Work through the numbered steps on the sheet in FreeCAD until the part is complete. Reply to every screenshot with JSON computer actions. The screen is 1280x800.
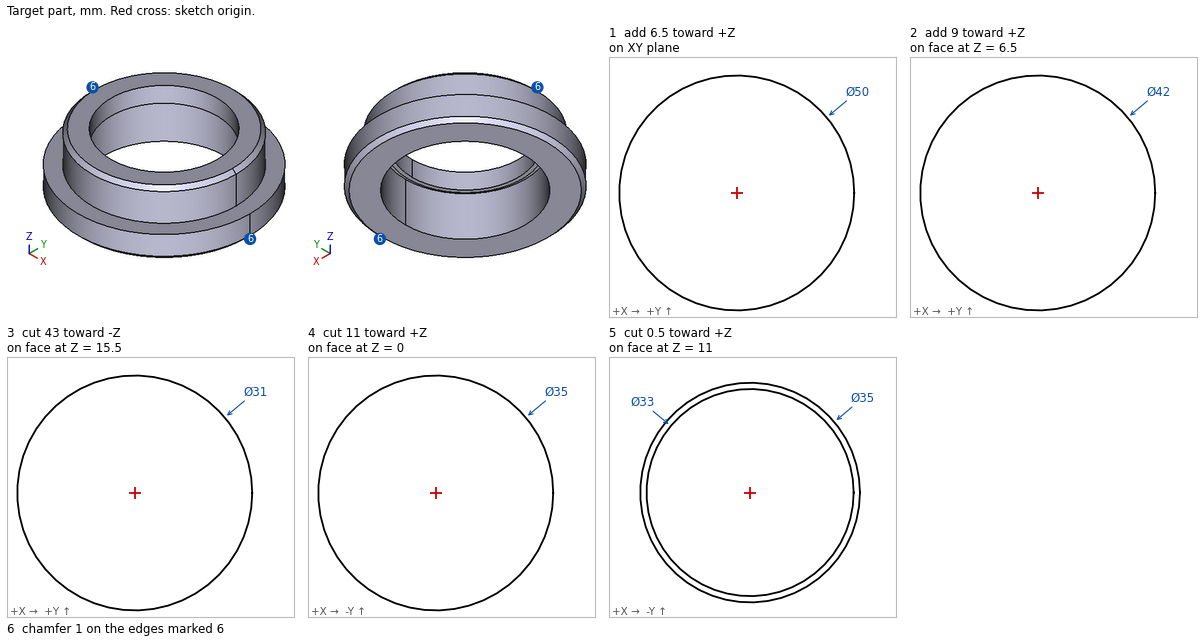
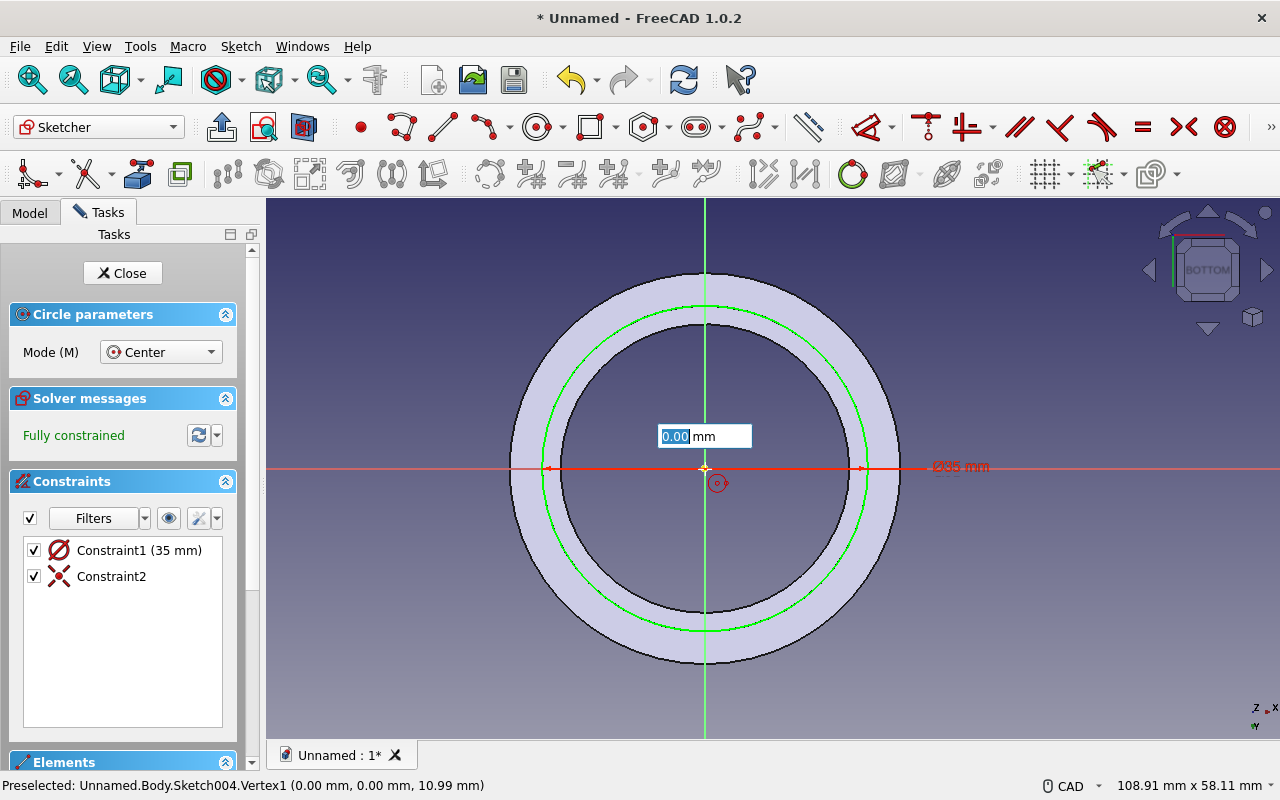
{"action": "scroll", "coordinate": [814, 360], "scroll_direction": "up", "scroll_amount": 3}
{"action": "mouse_move", "coordinate": [813, 360]}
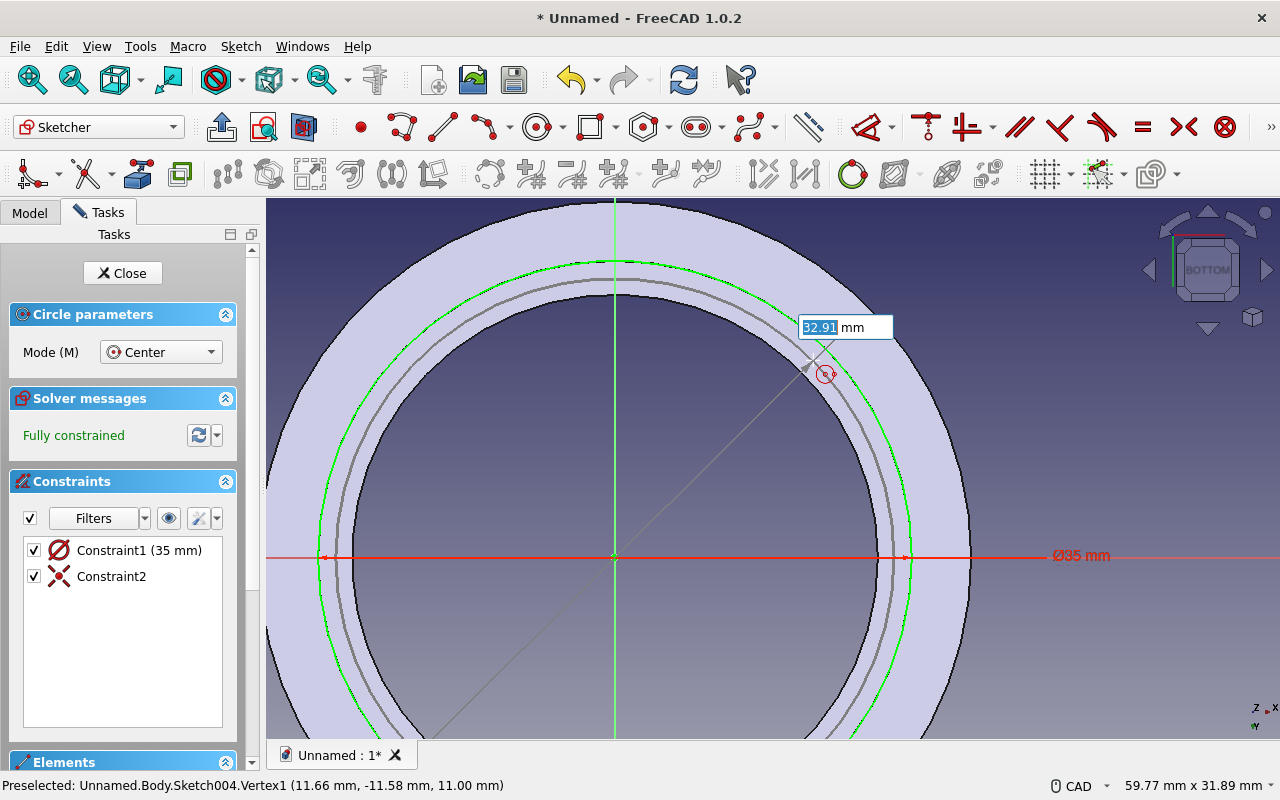
{"action": "type", "text": "33"}
{"action": "key", "text": "Return"}
{"action": "key", "text": "Escape"}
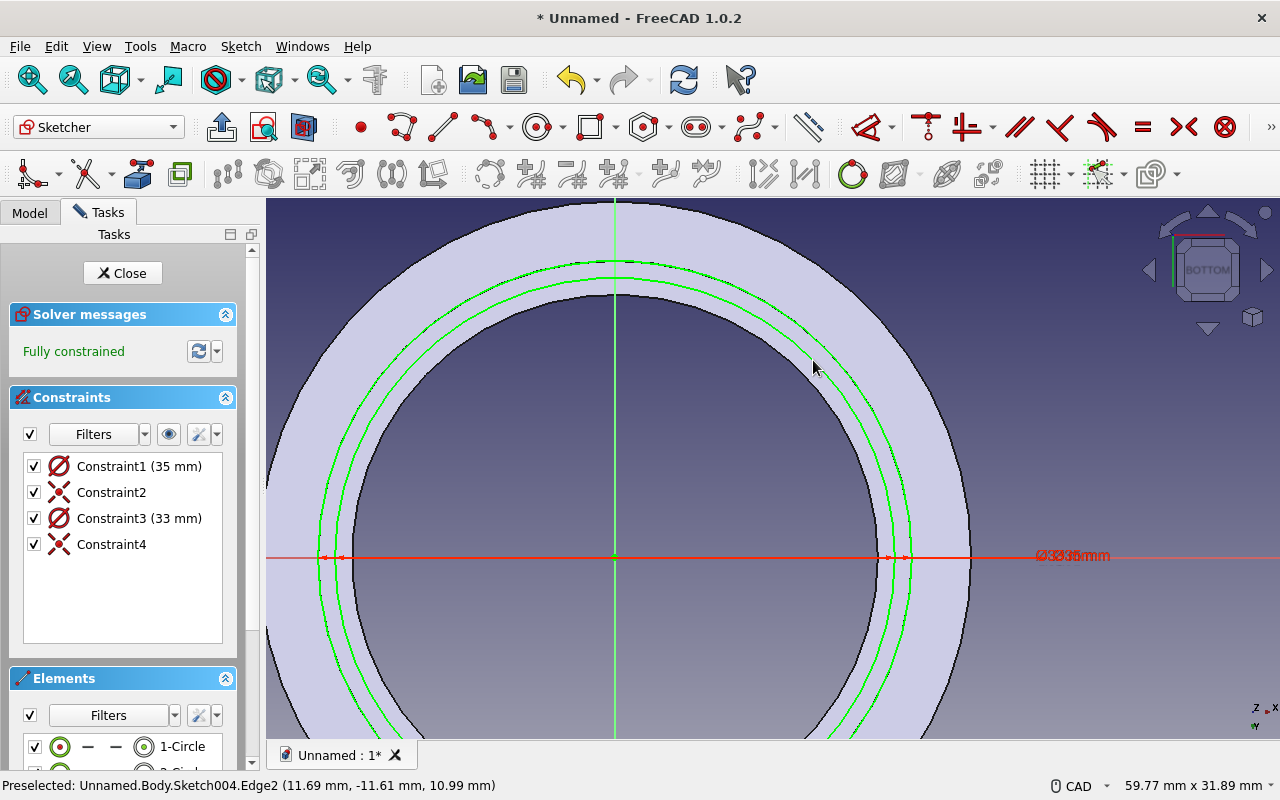
{"action": "left_click", "coordinate": [123, 273]}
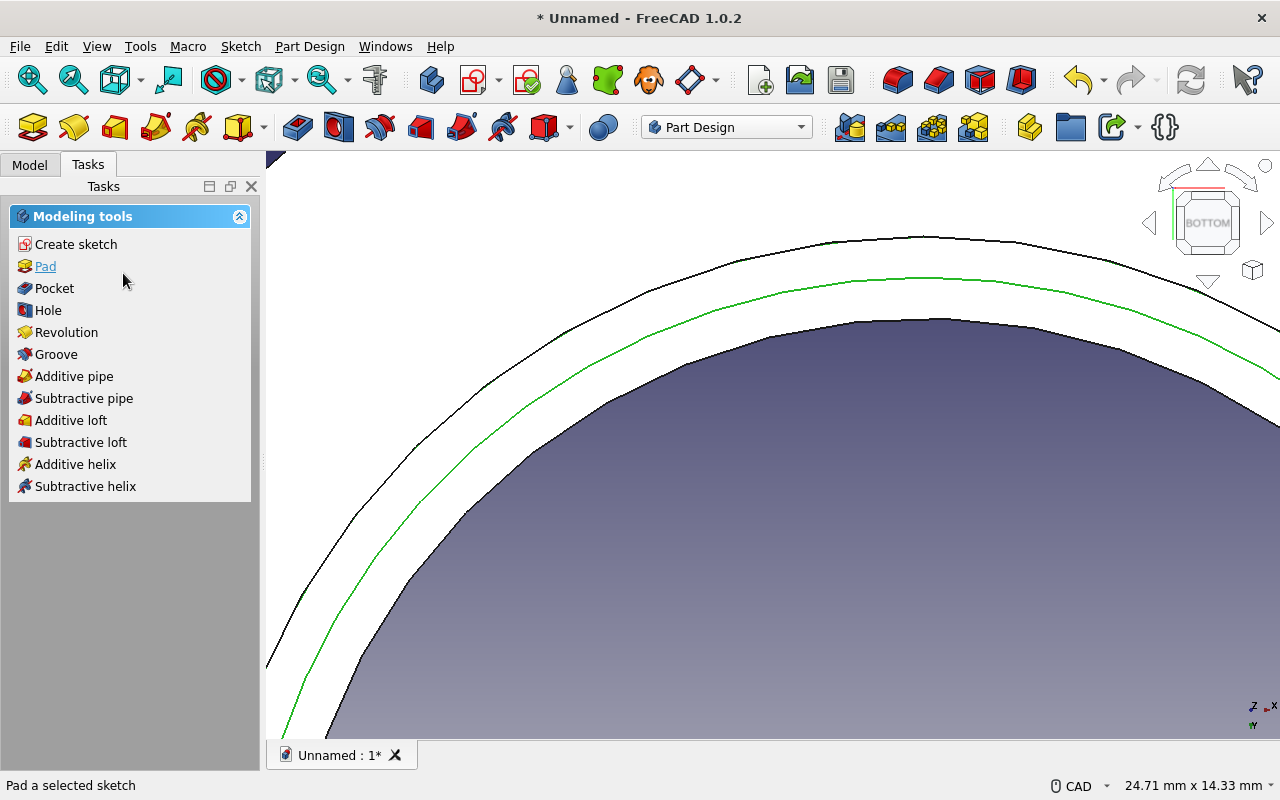
{"action": "left_click", "coordinate": [298, 128]}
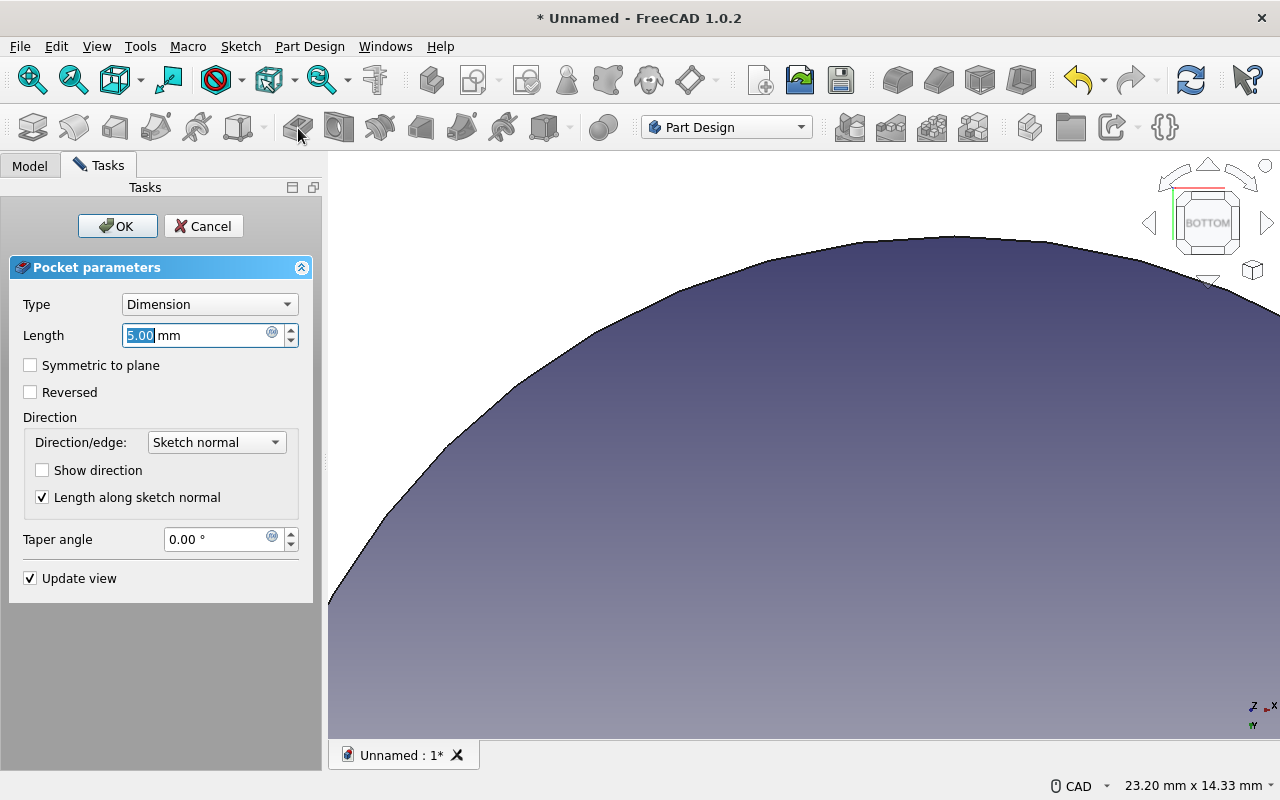
{"action": "type", "text": "0.5"}
{"action": "key", "text": "Tab"}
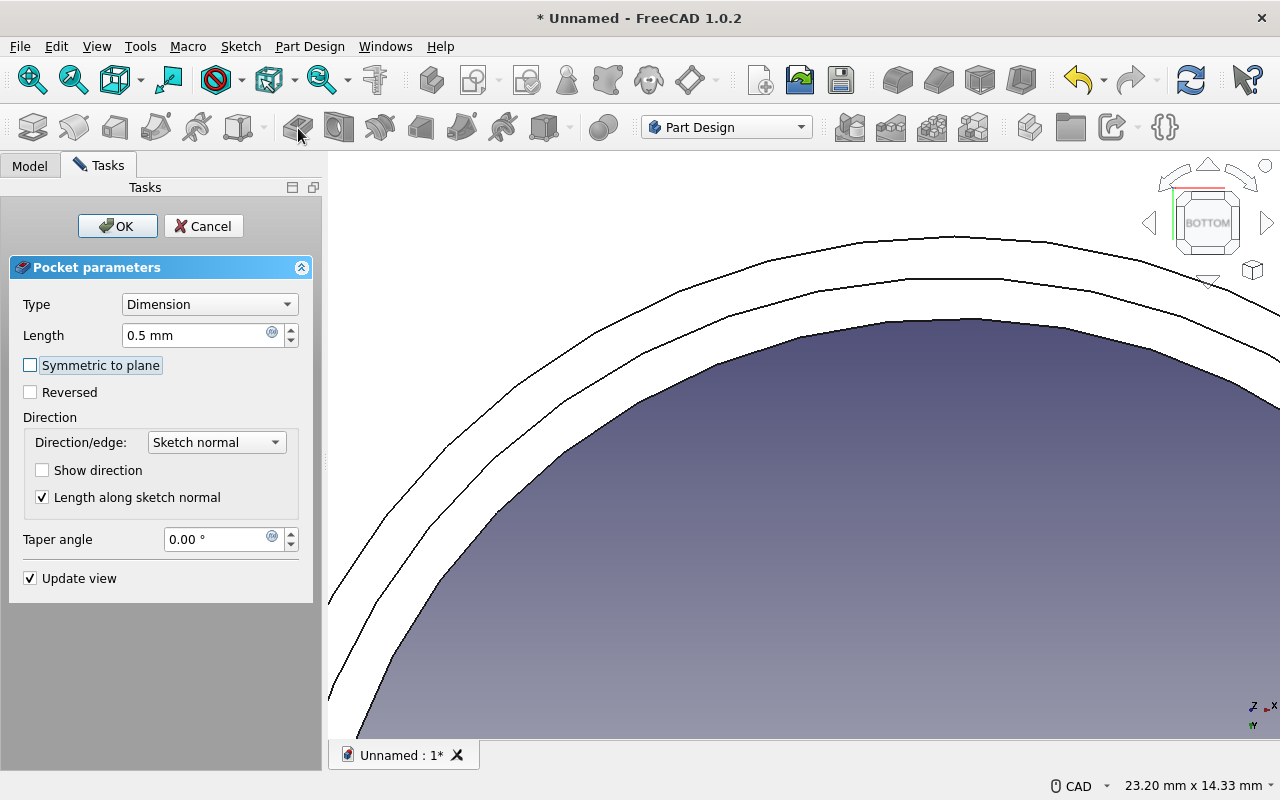
{"action": "left_click", "coordinate": [118, 226]}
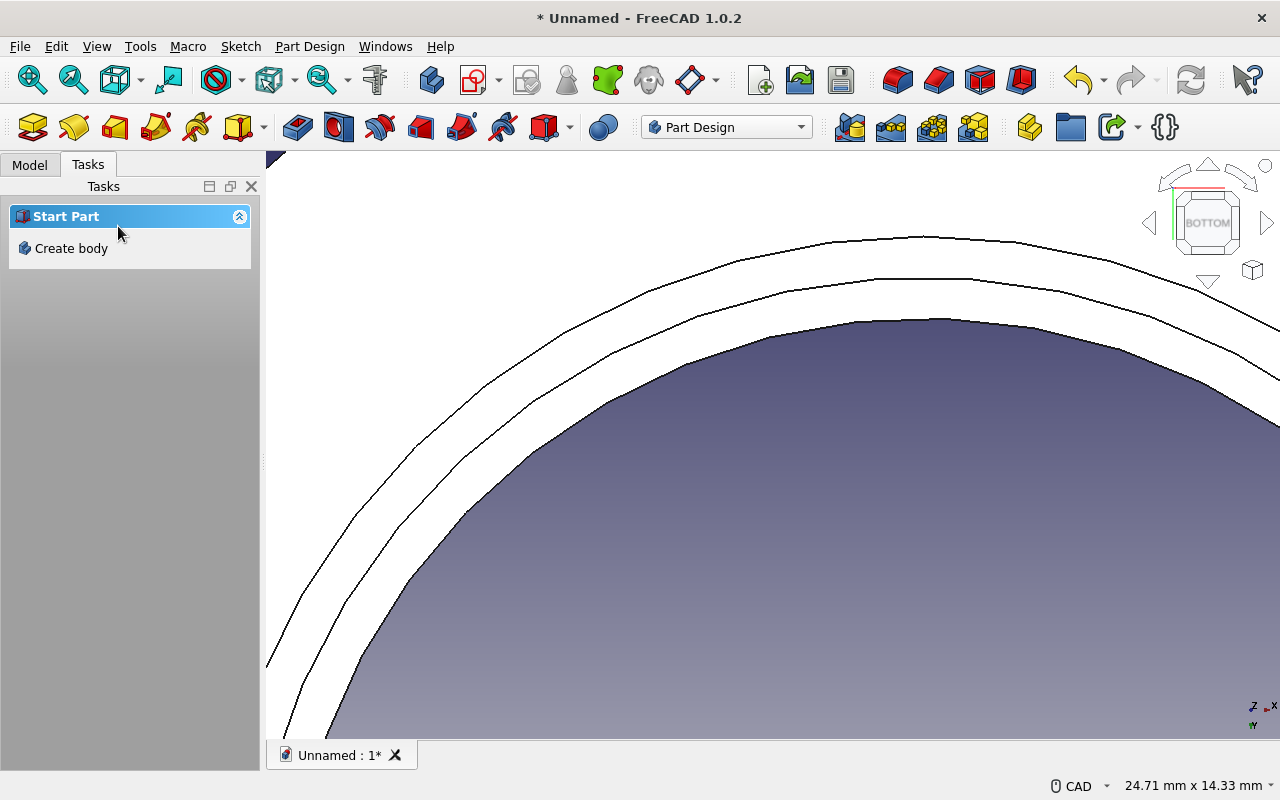
{"action": "left_click", "coordinate": [33, 80]}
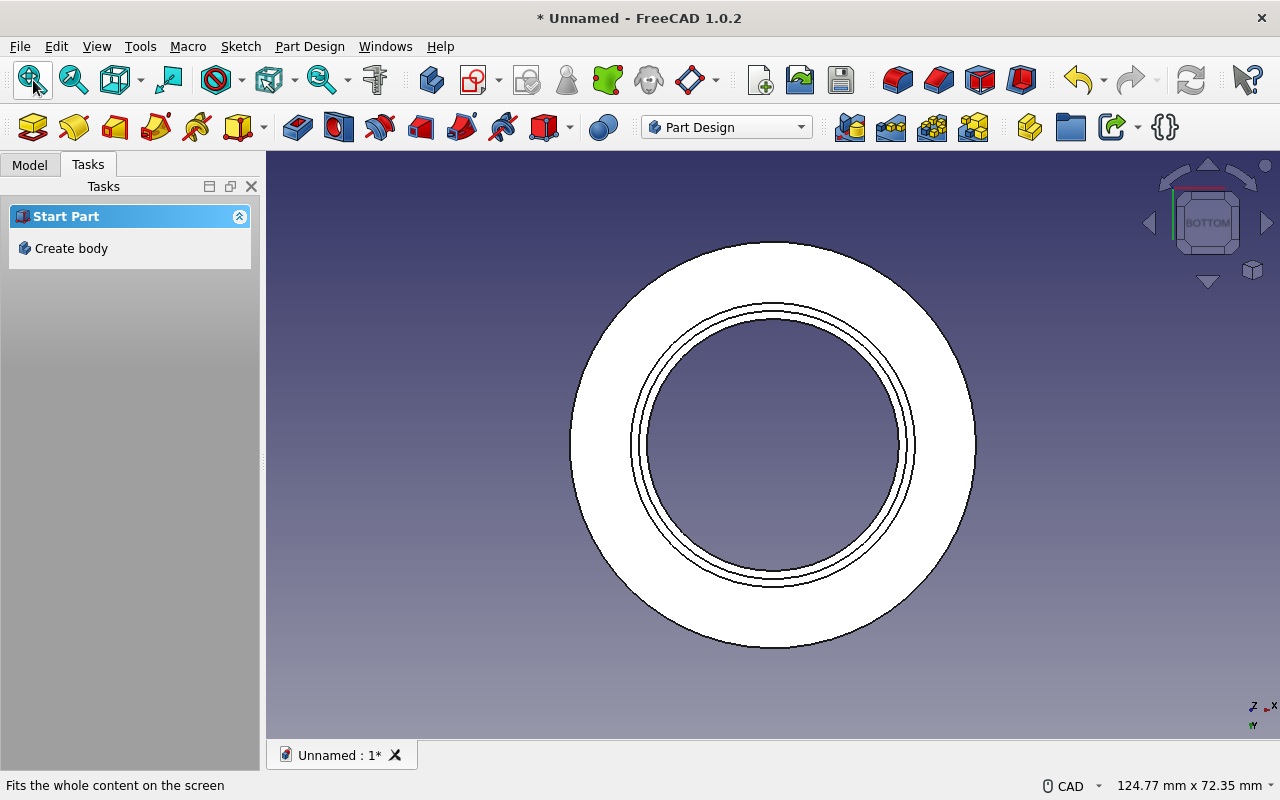
{"action": "left_click", "coordinate": [608, 563]}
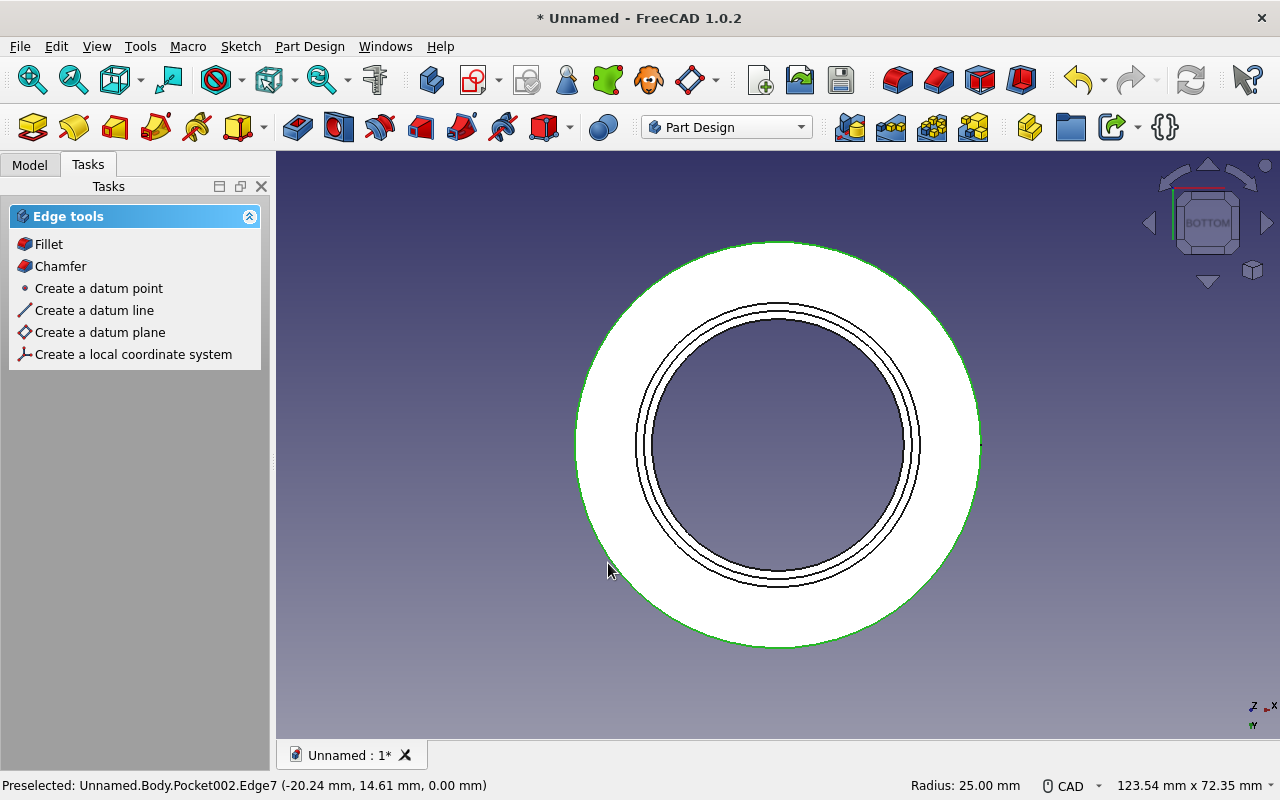
{"action": "key", "text": "0"}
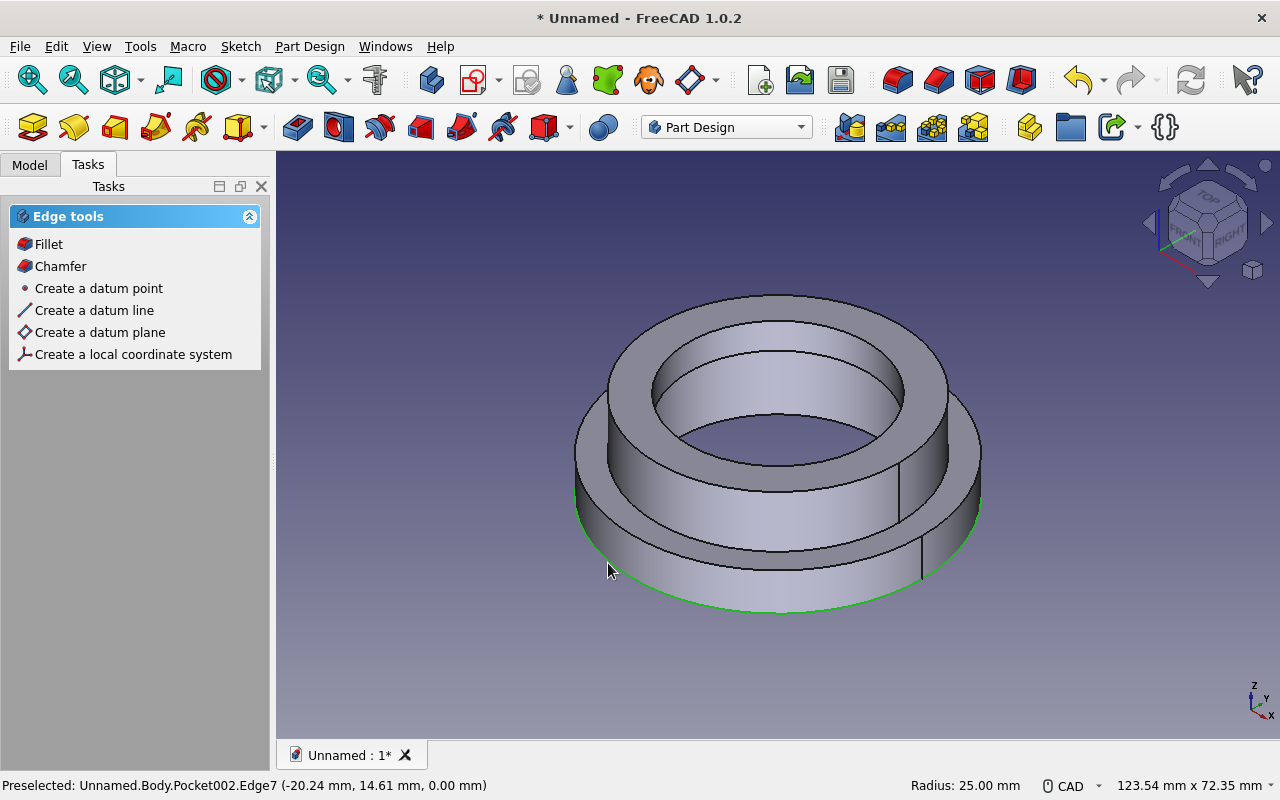
{"action": "left_click", "coordinate": [626, 437], "text": "ctrl"}